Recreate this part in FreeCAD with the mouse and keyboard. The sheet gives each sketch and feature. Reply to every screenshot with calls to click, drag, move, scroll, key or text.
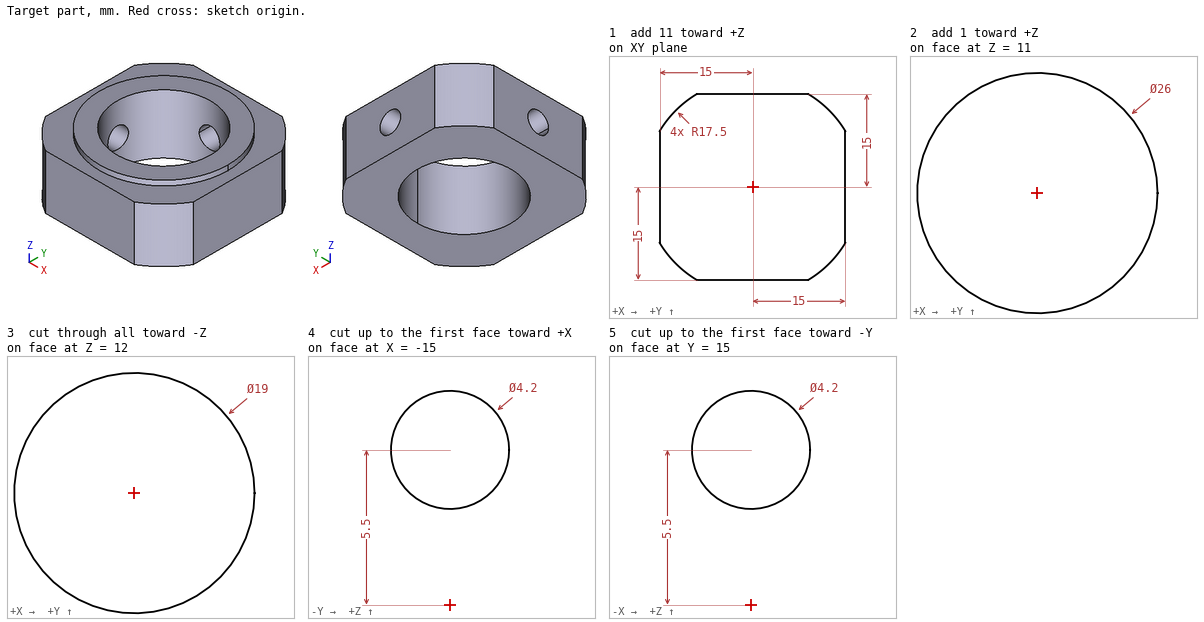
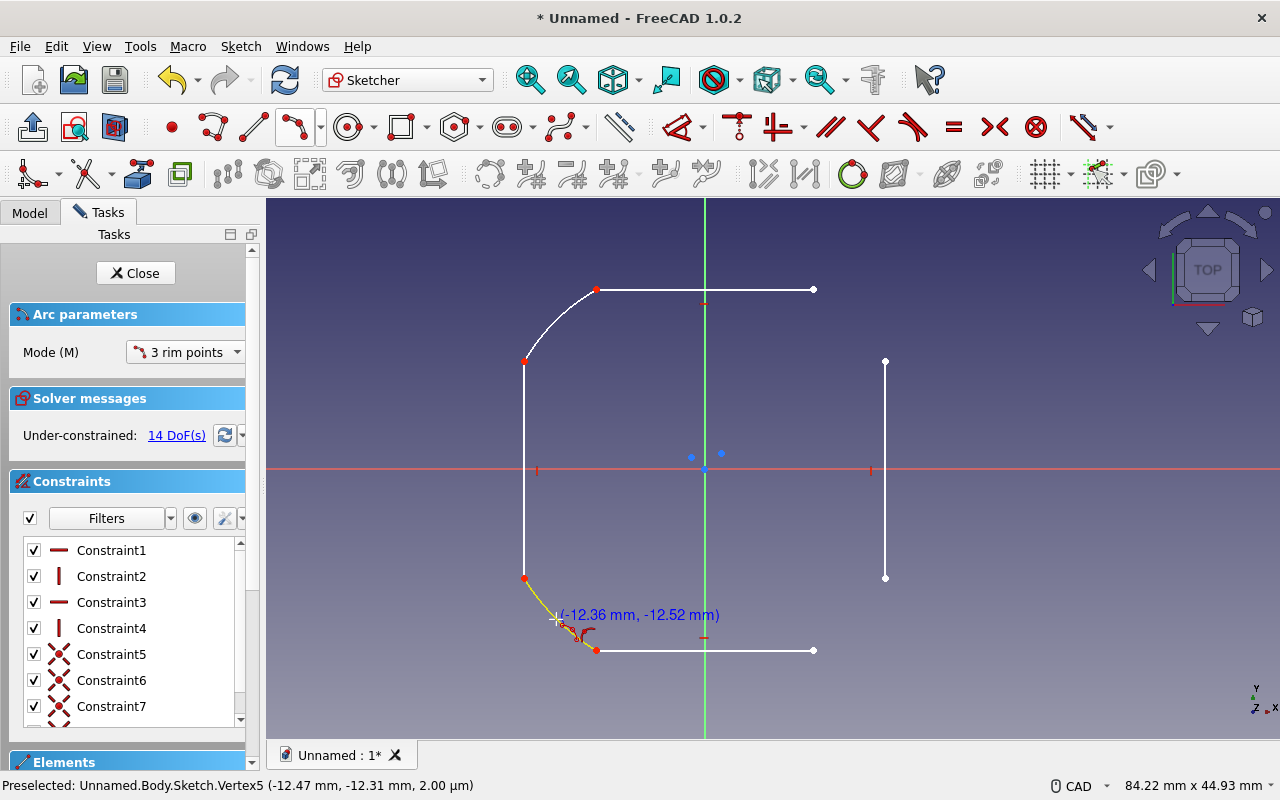
click(813, 651)
click(885, 579)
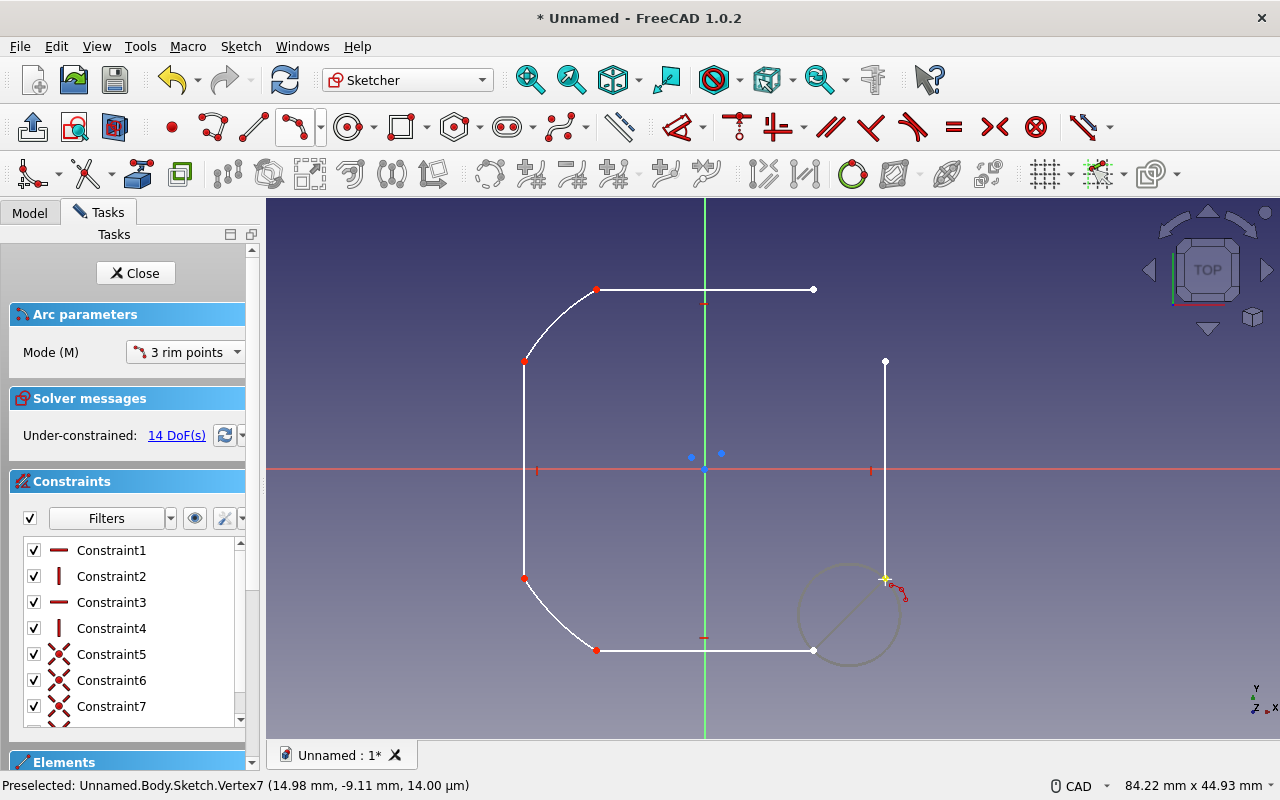
scroll(854, 618, up, 5)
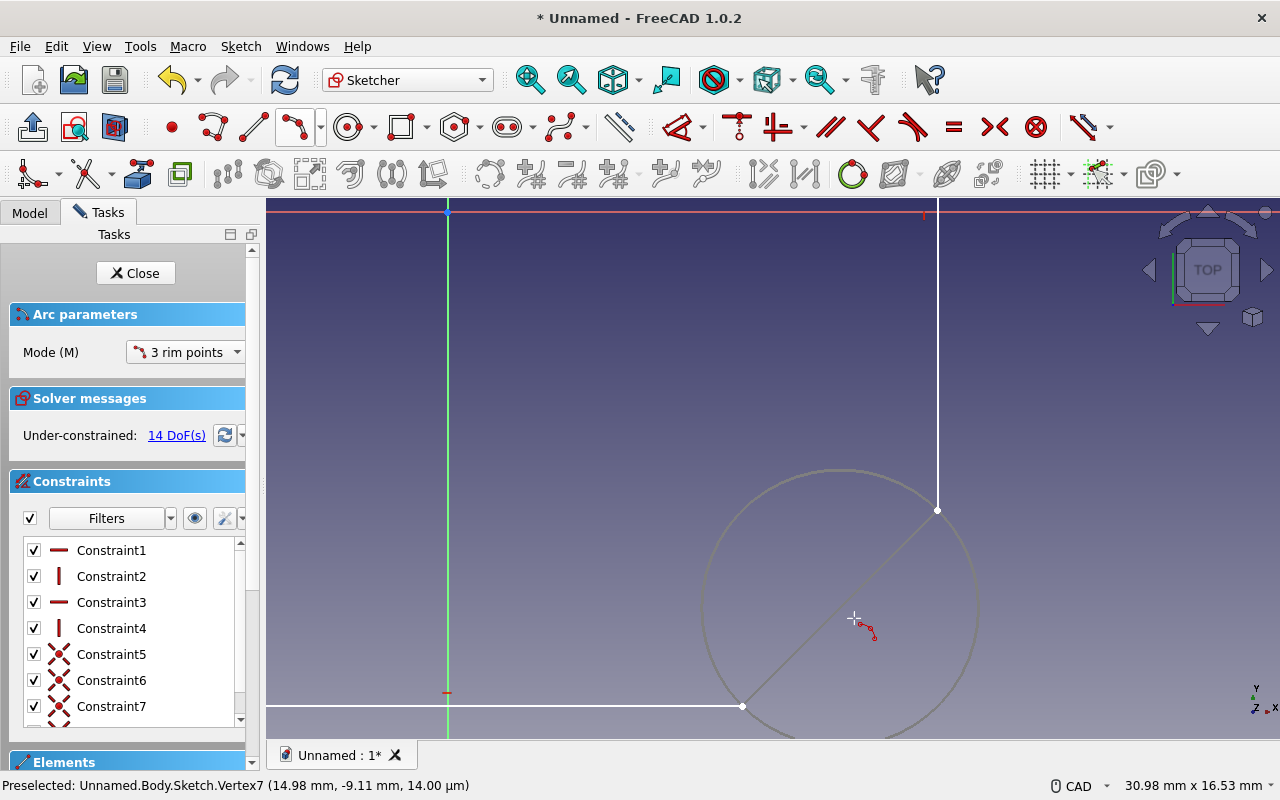
click(853, 617)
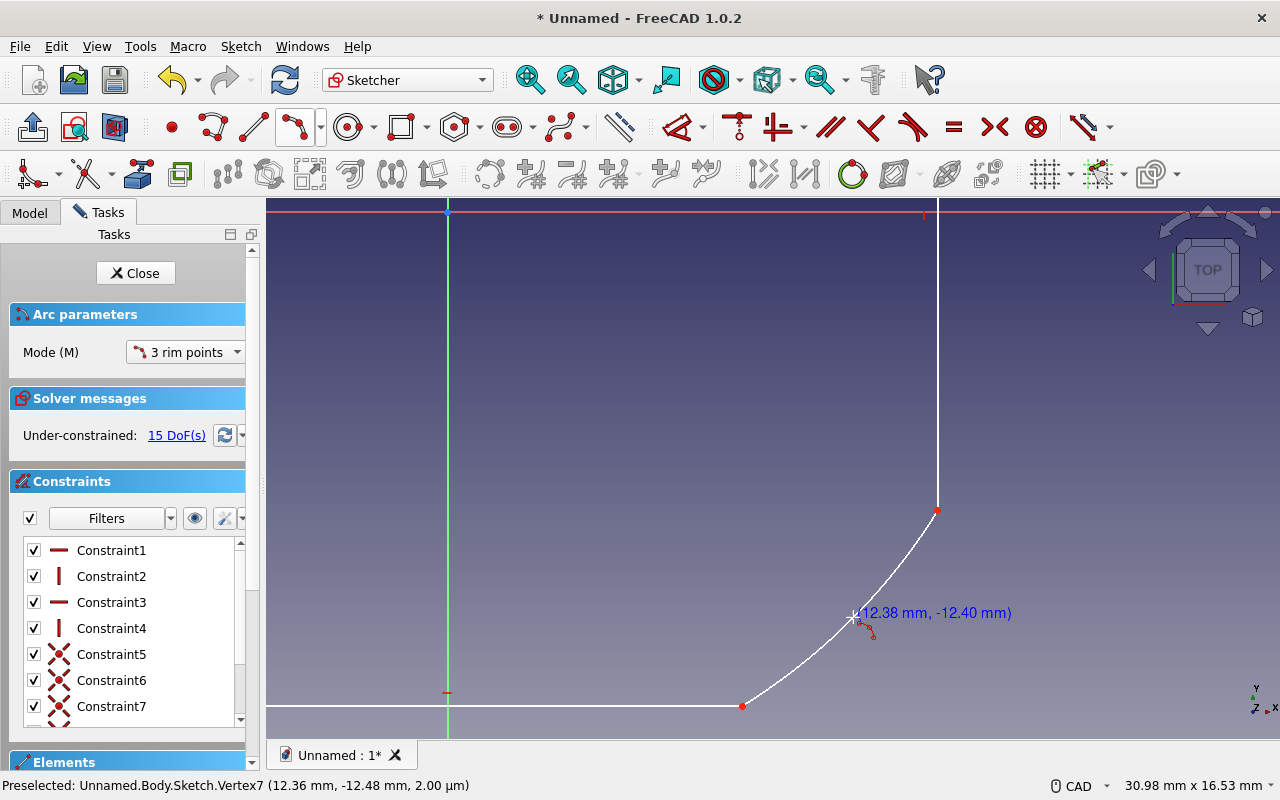
scroll(854, 618, down, 5)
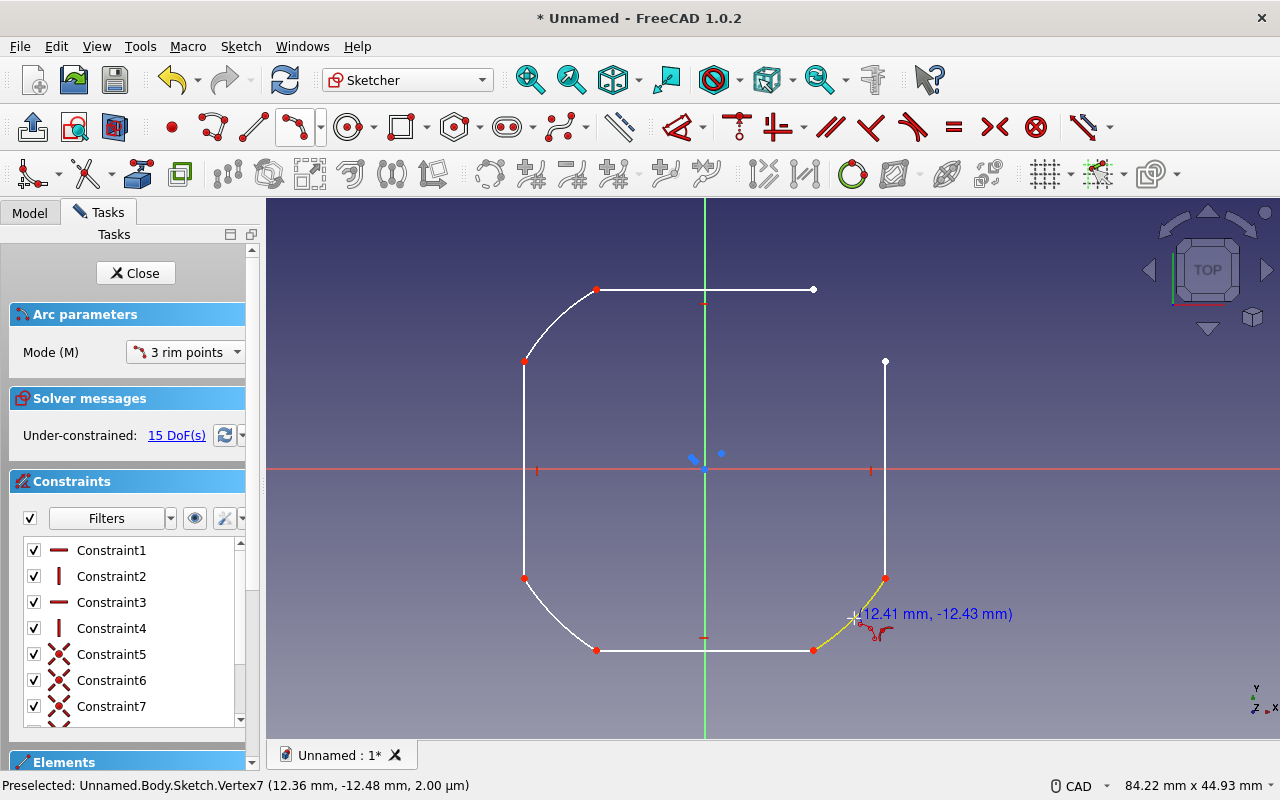
click(885, 362)
click(813, 290)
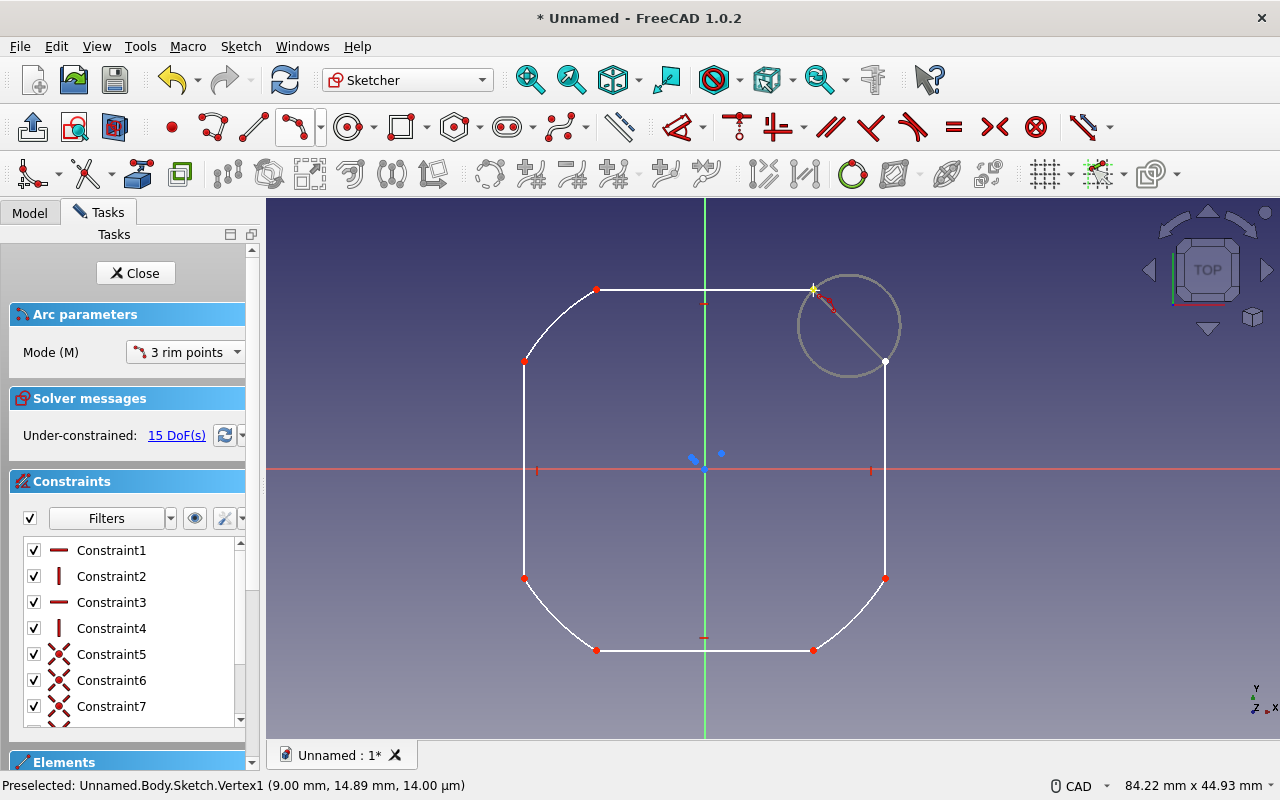
scroll(854, 320, up, 5)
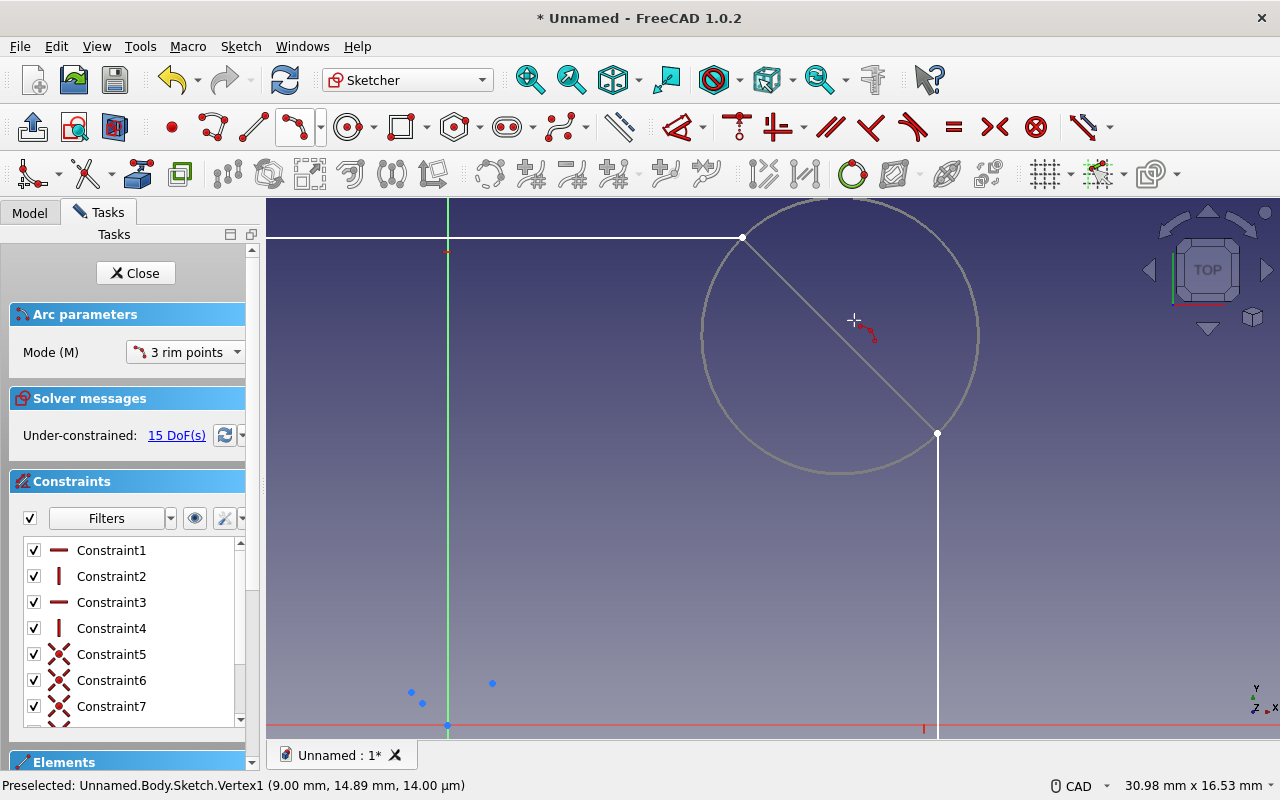
click(853, 320)
key(Escape)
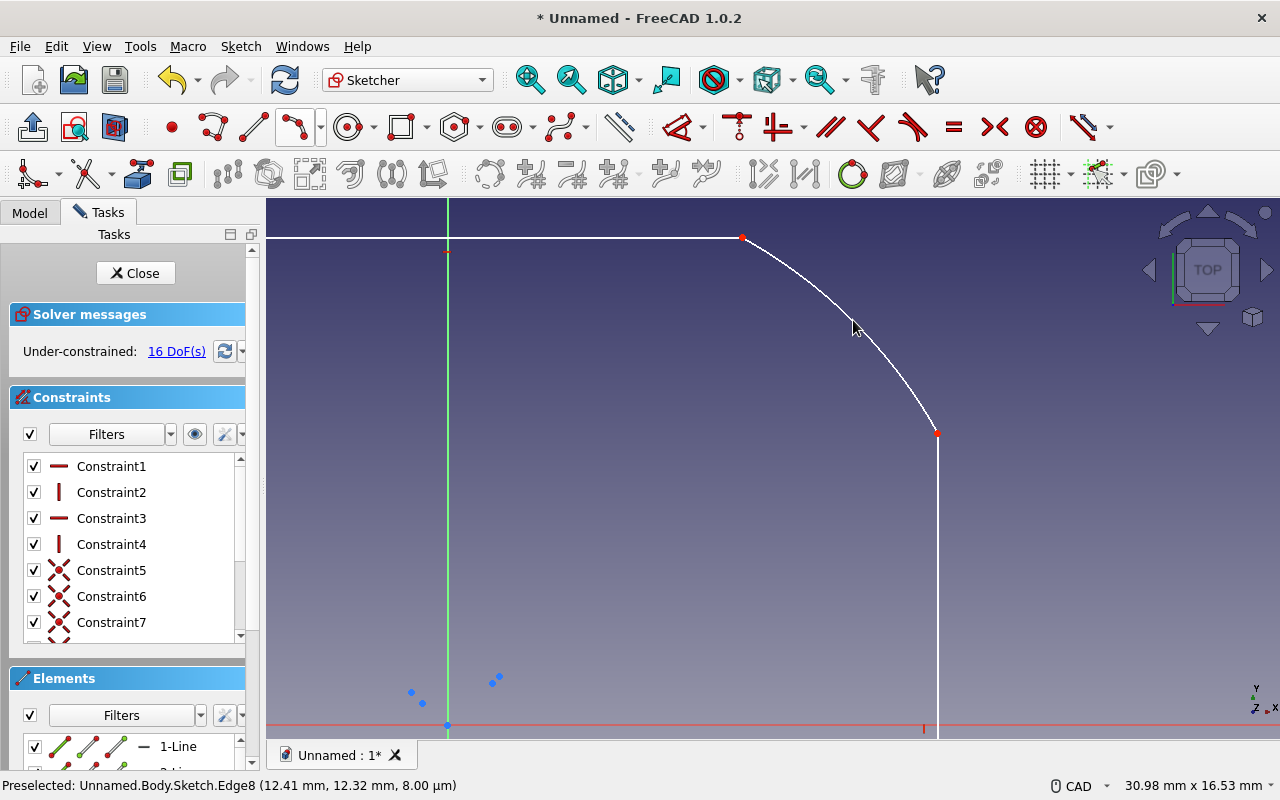
scroll(854, 319, down, 5)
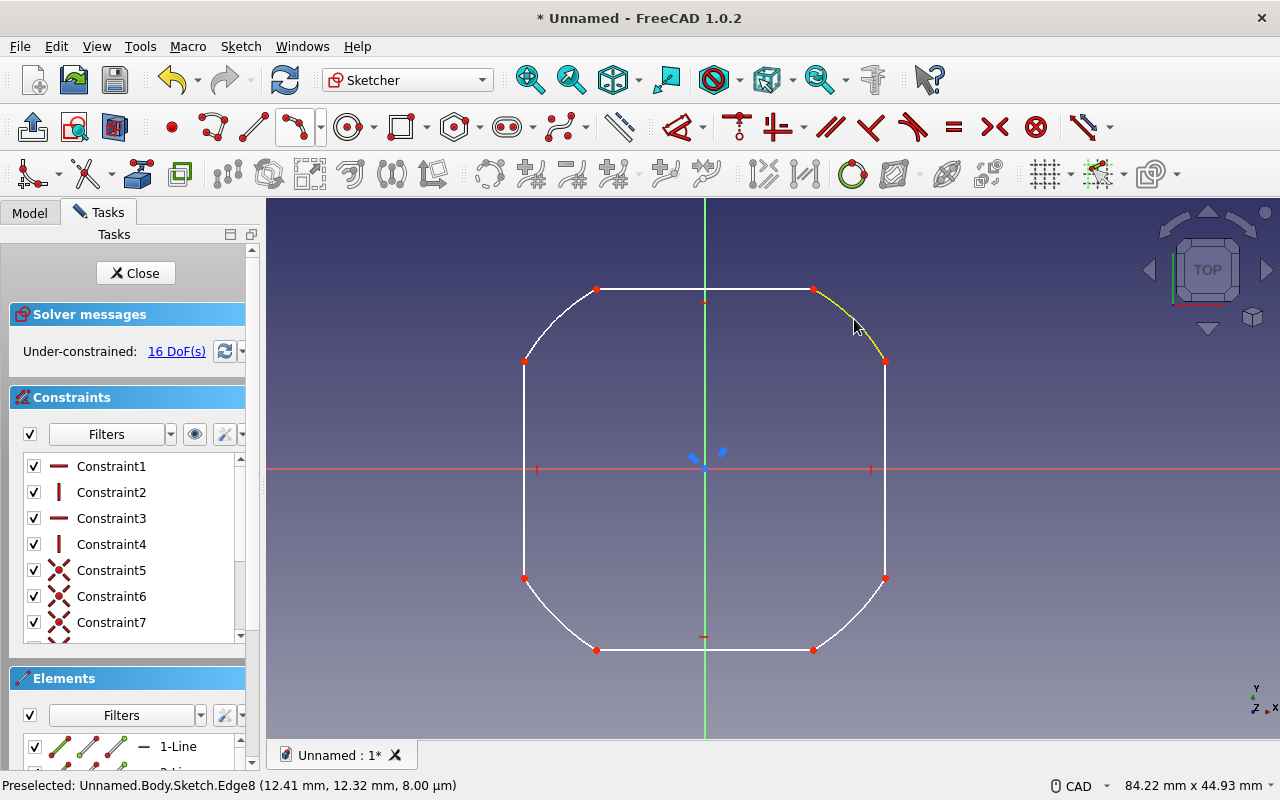
click(571, 307)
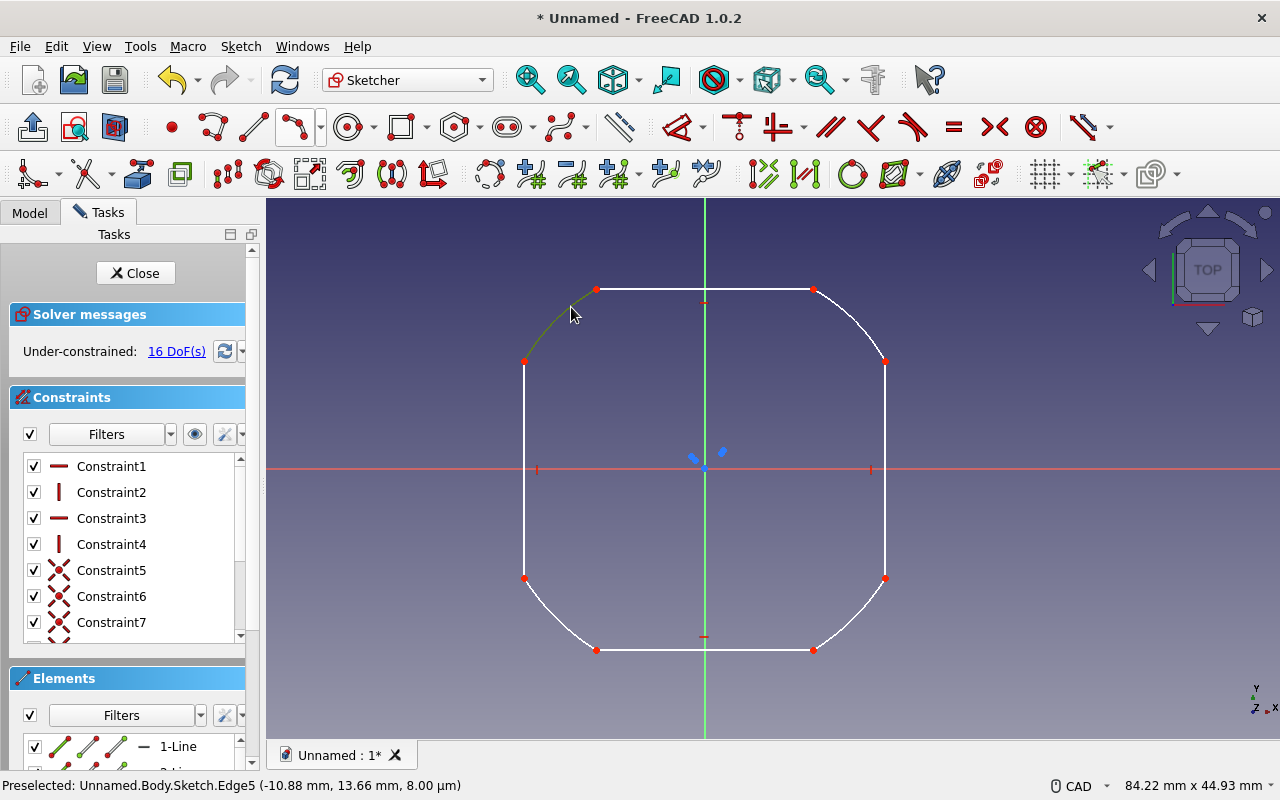
click(542, 603)